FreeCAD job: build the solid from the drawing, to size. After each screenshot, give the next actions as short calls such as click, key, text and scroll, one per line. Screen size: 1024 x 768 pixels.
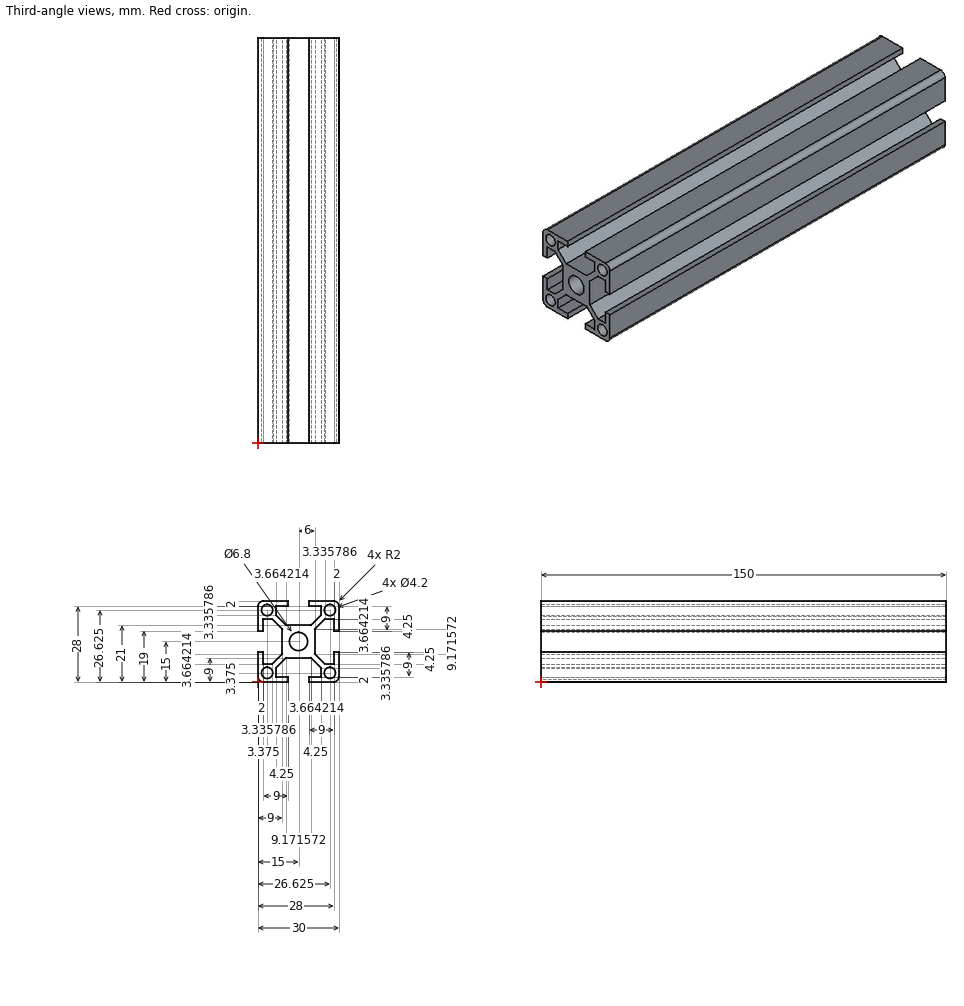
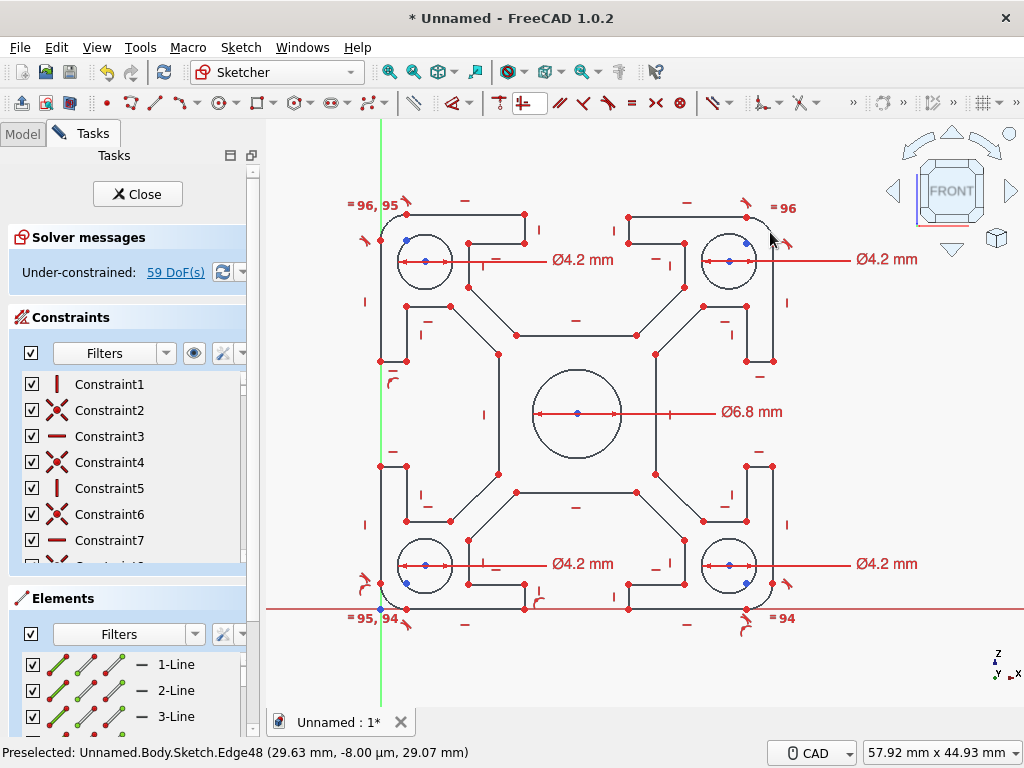
click(452, 104)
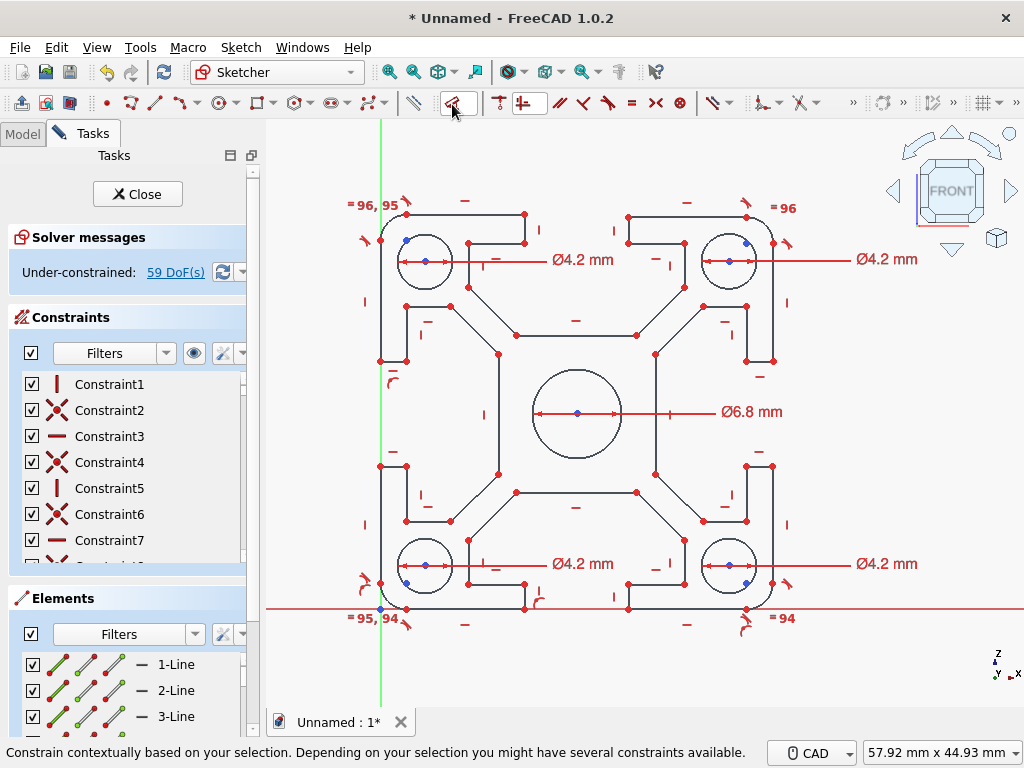
scroll(758, 606, up, 3)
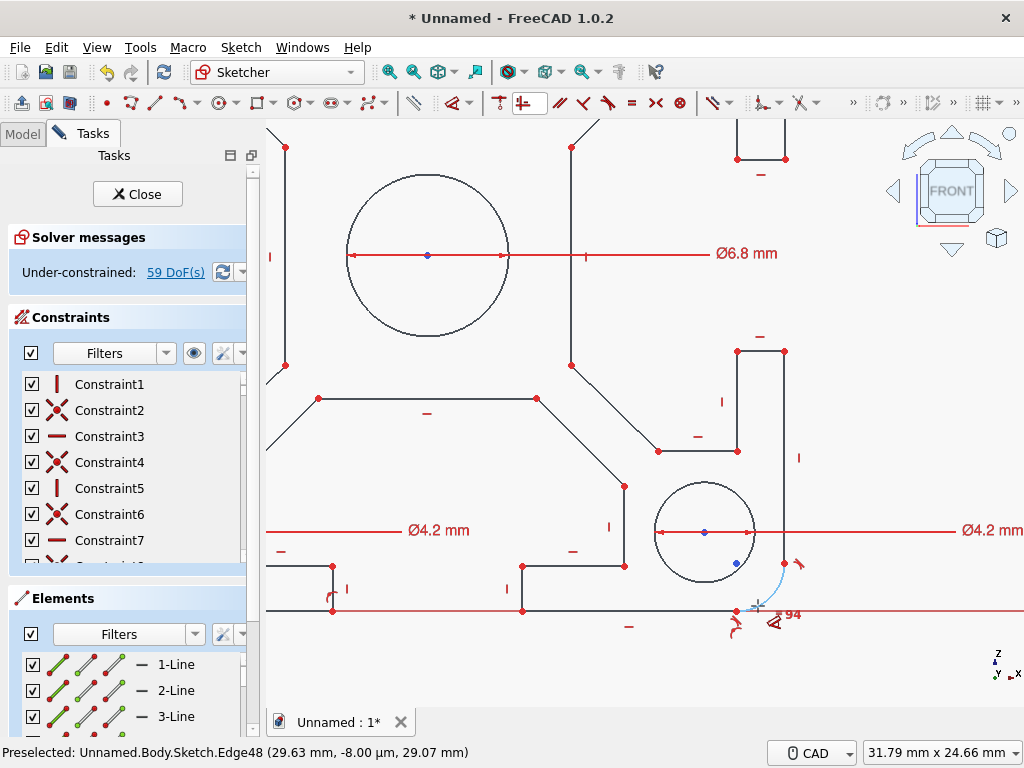
click(758, 606)
click(772, 635)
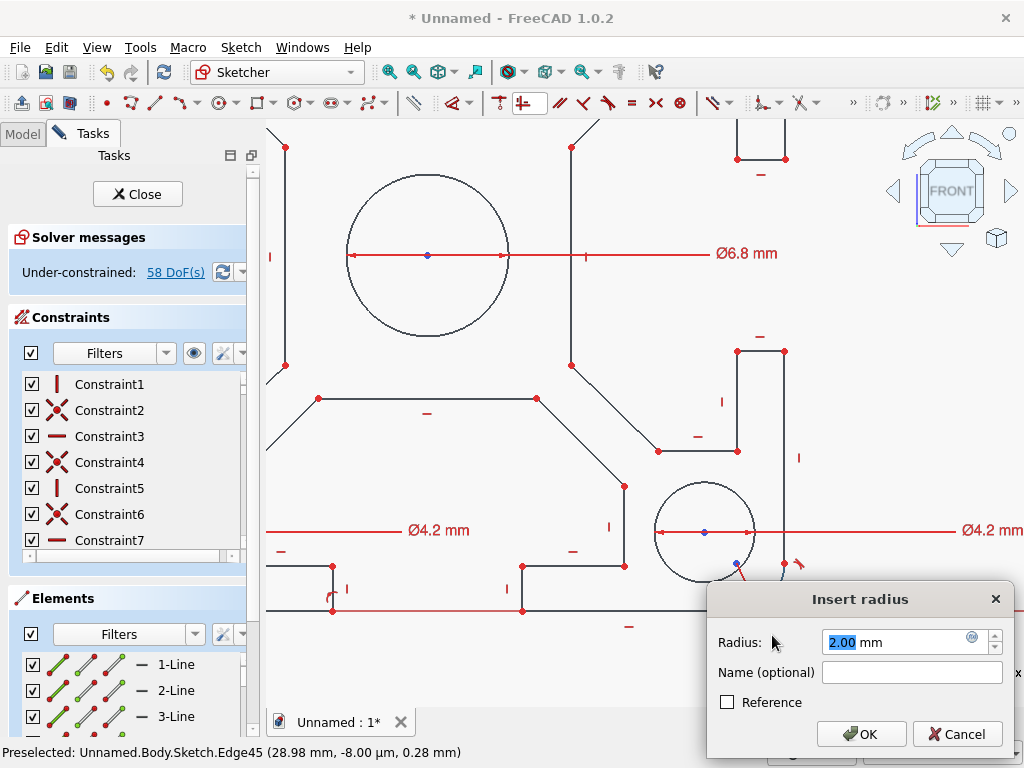
text(2)
key(Return)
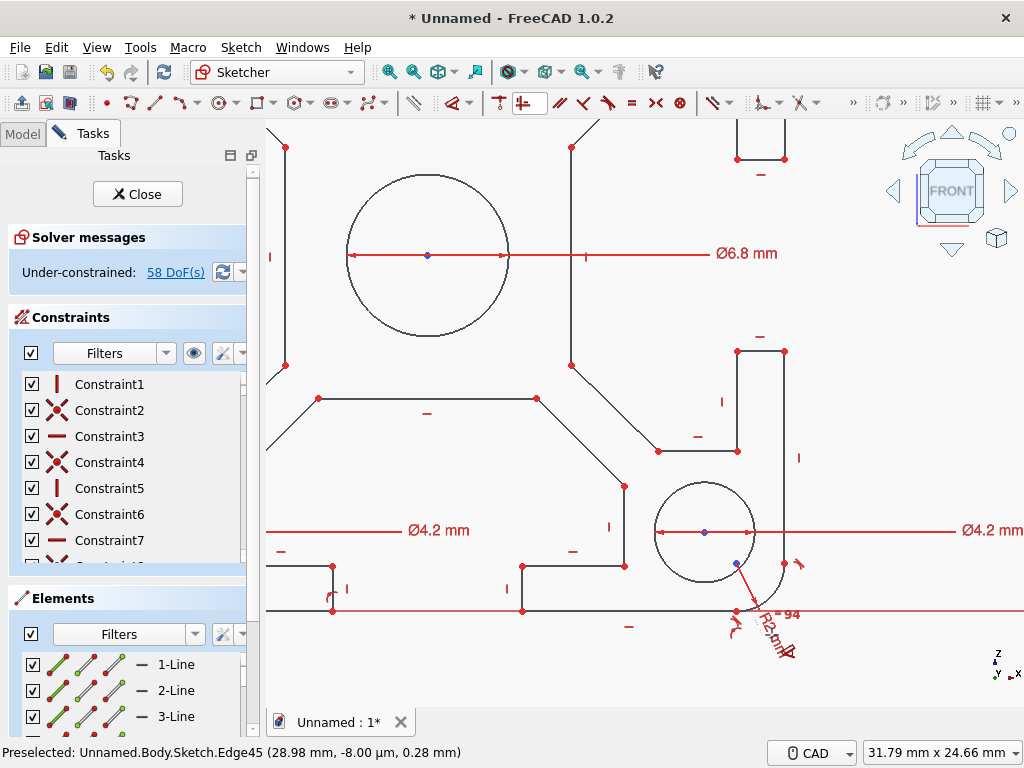
scroll(758, 607, down, 3)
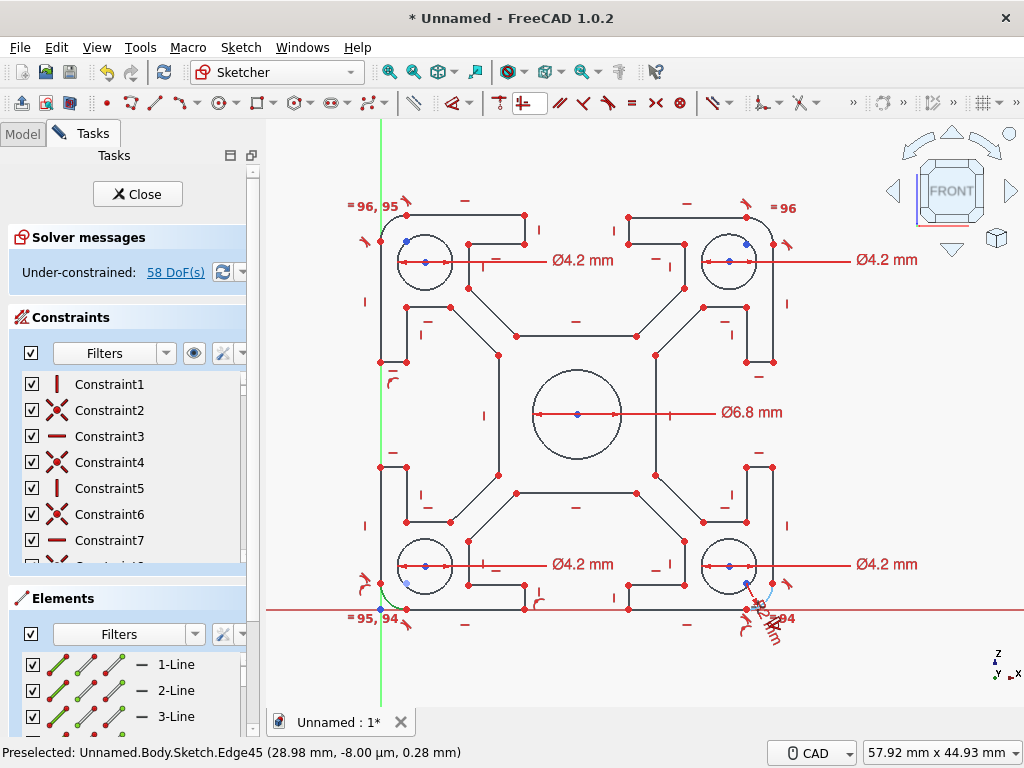
click(773, 279)
click(807, 303)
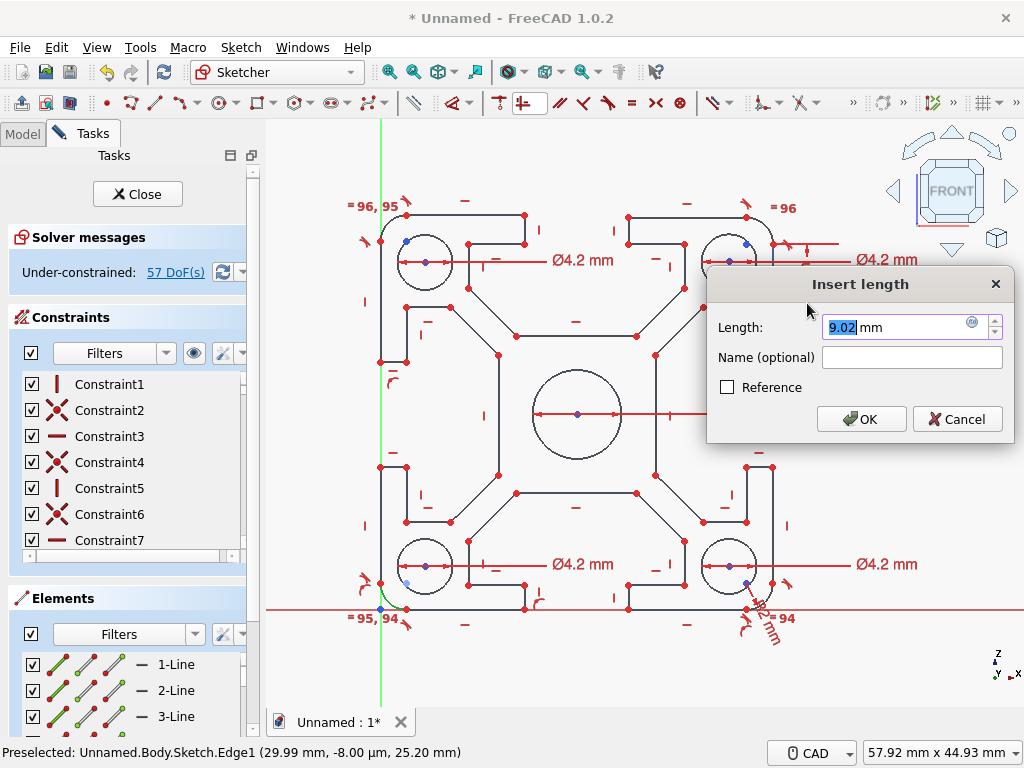
text(9)
key(Return)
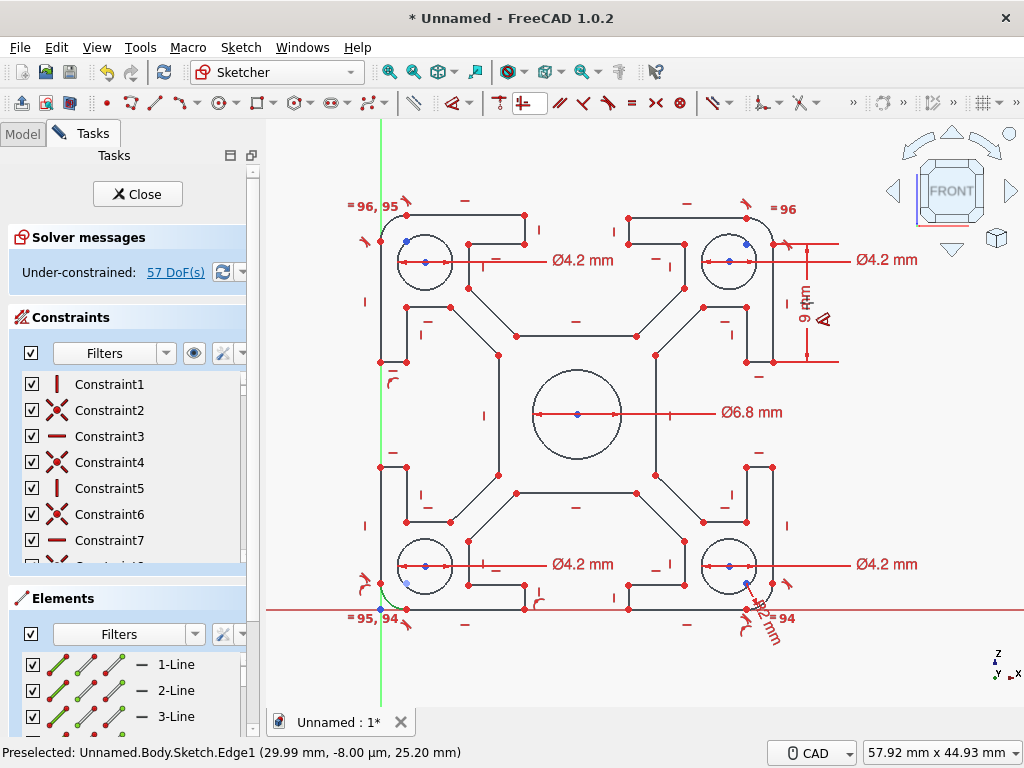
scroll(763, 362, up, 3)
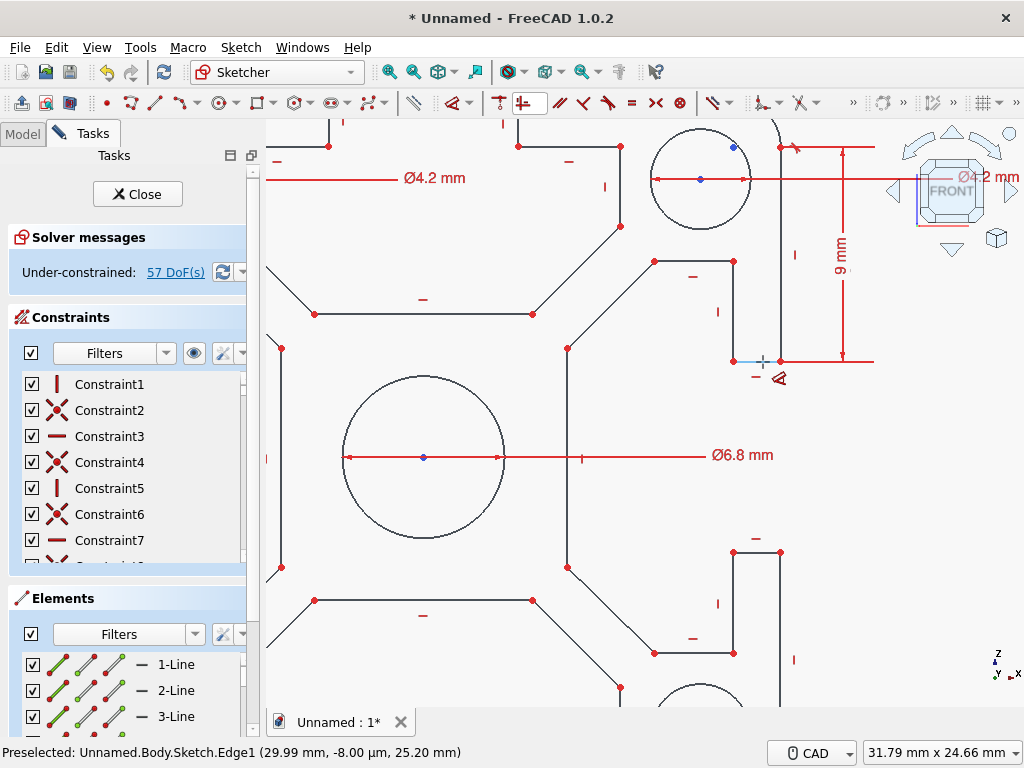
click(762, 362)
click(757, 328)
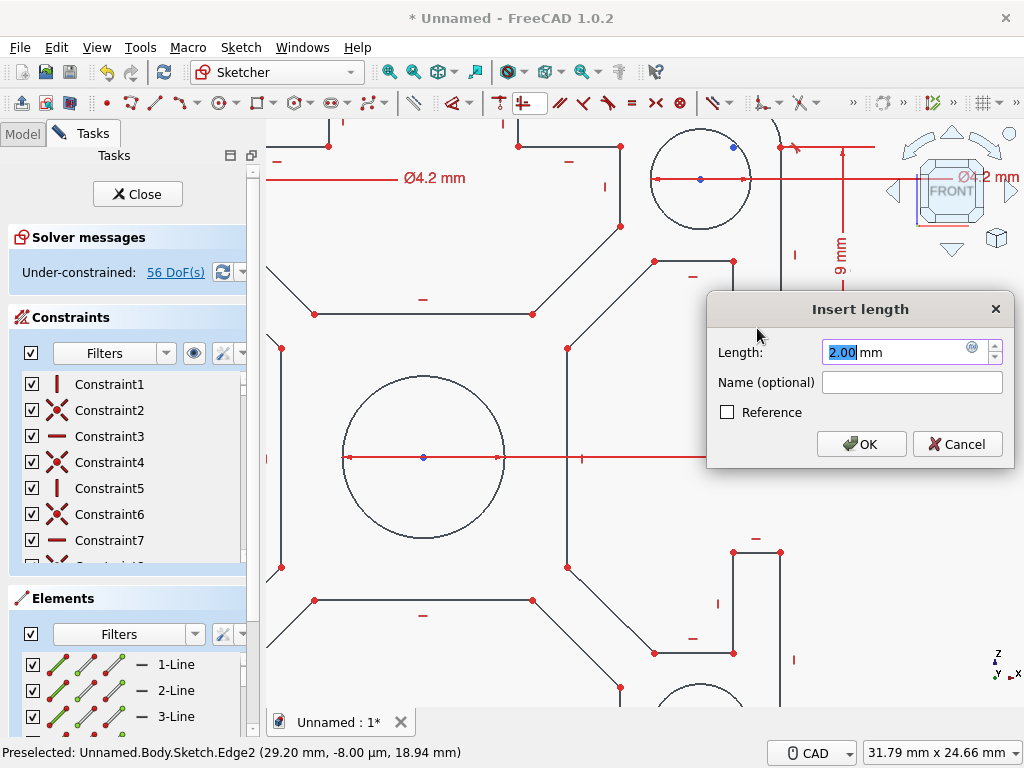
text(2)
key(Return)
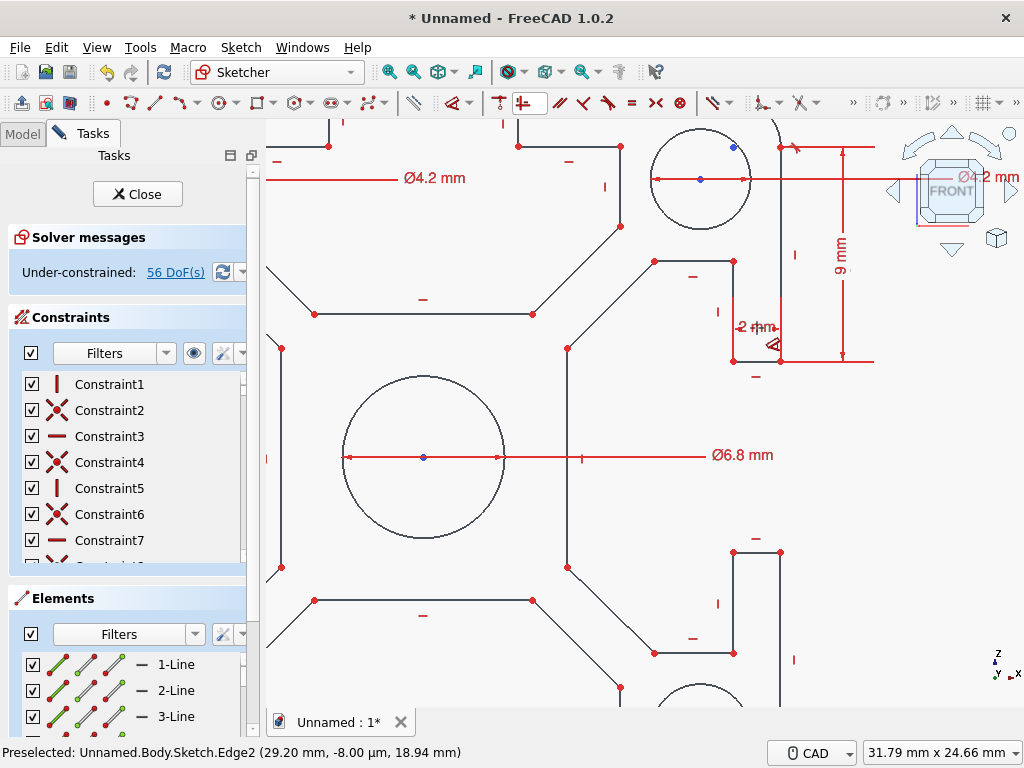
click(747, 553)
click(757, 587)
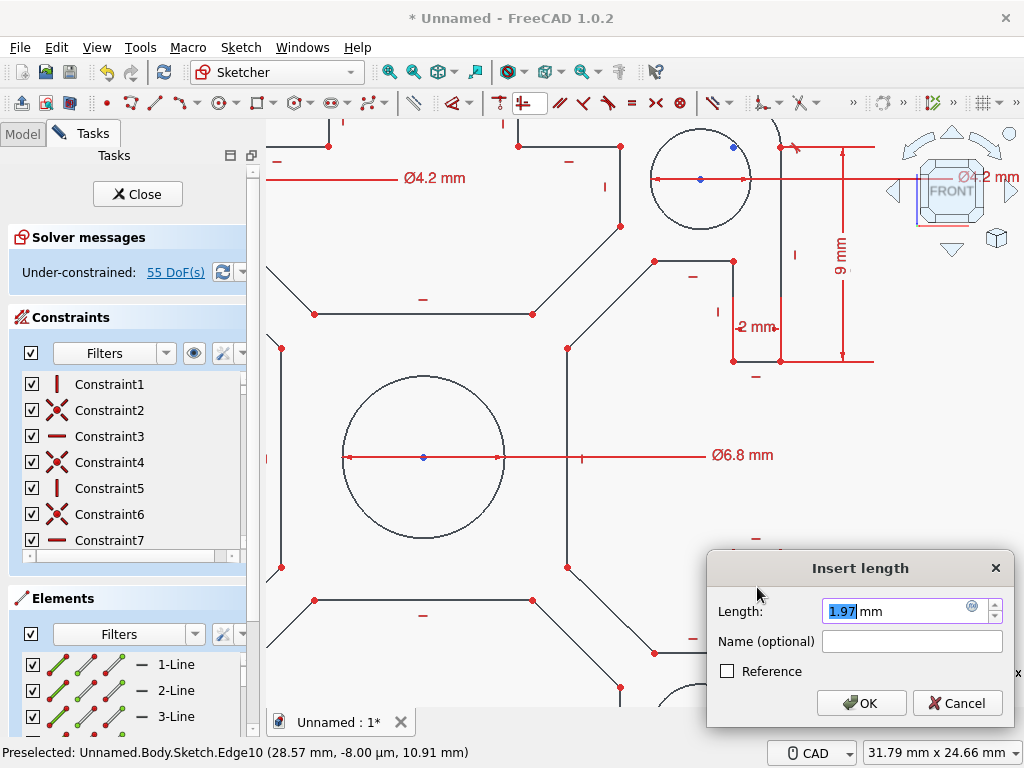
text(2)
key(Return)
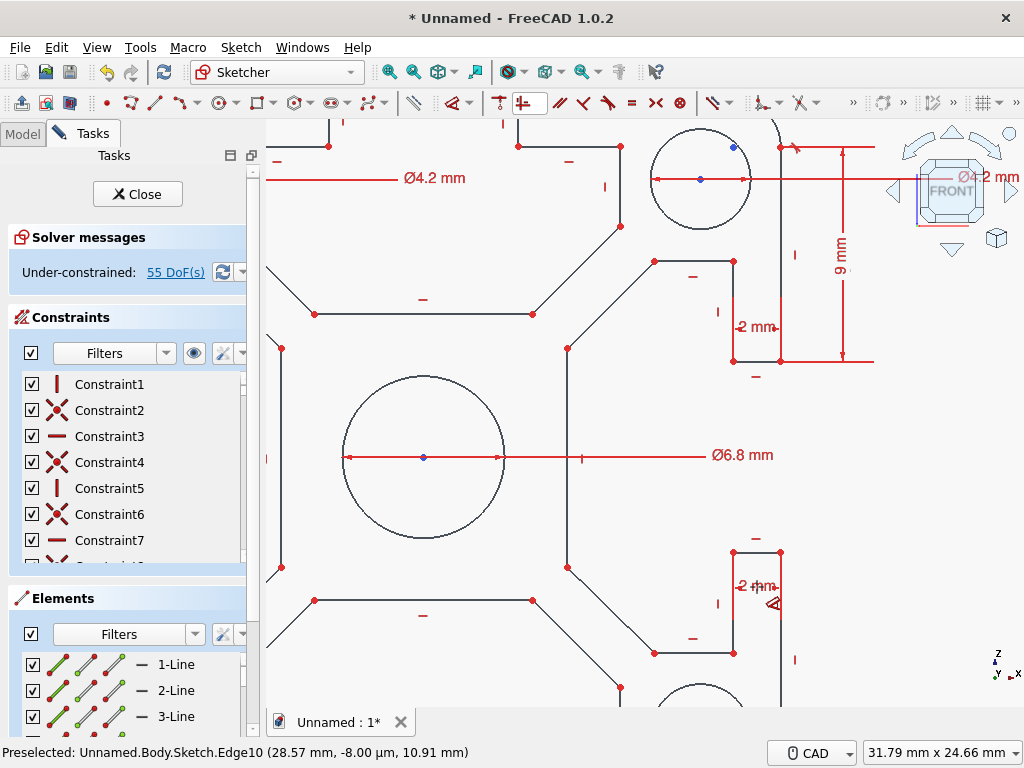
click(781, 617)
click(815, 616)